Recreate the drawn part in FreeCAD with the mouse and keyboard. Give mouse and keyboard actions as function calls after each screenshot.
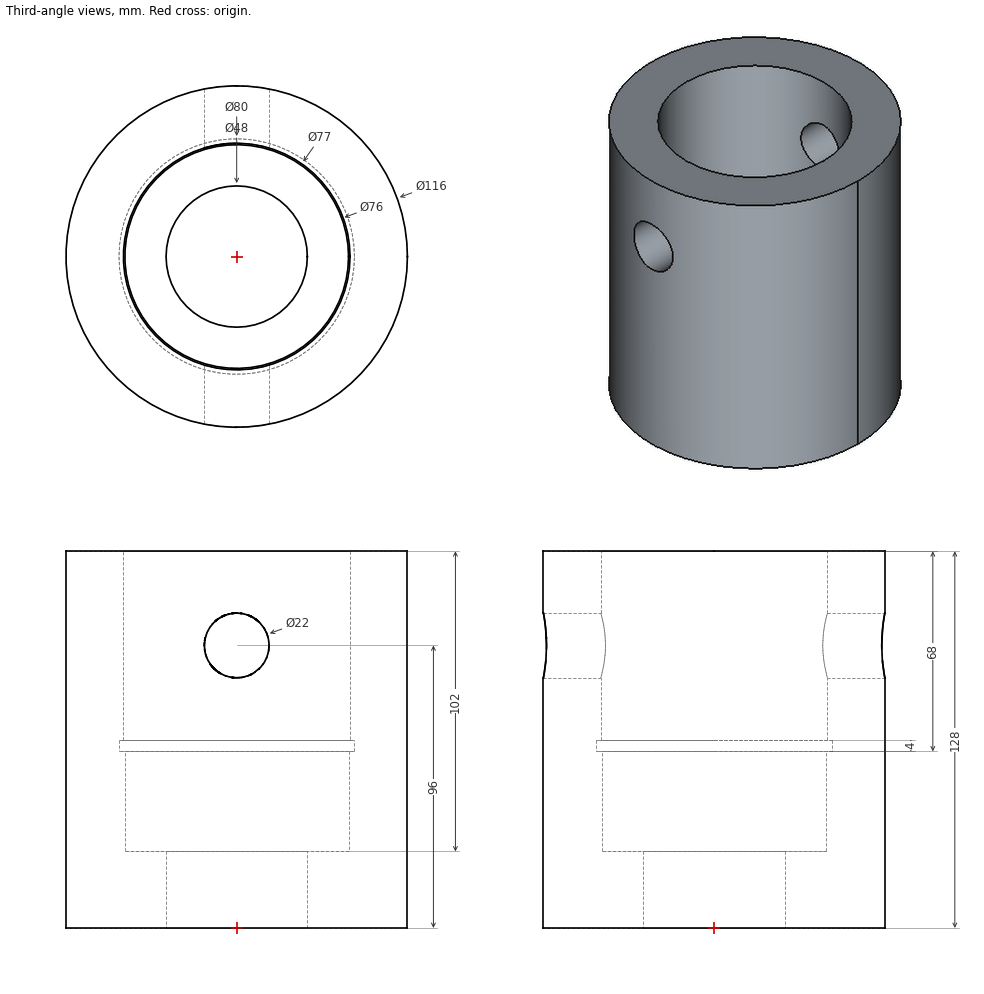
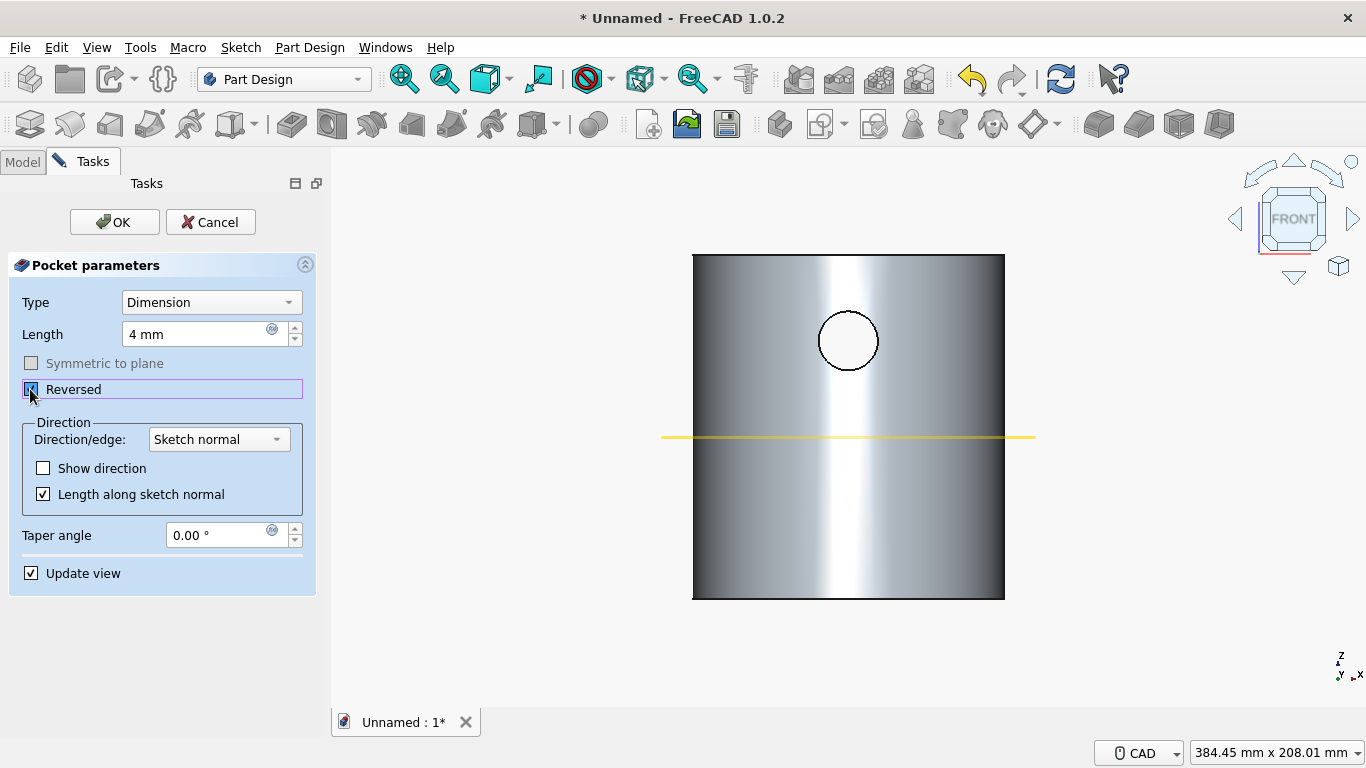
click(115, 222)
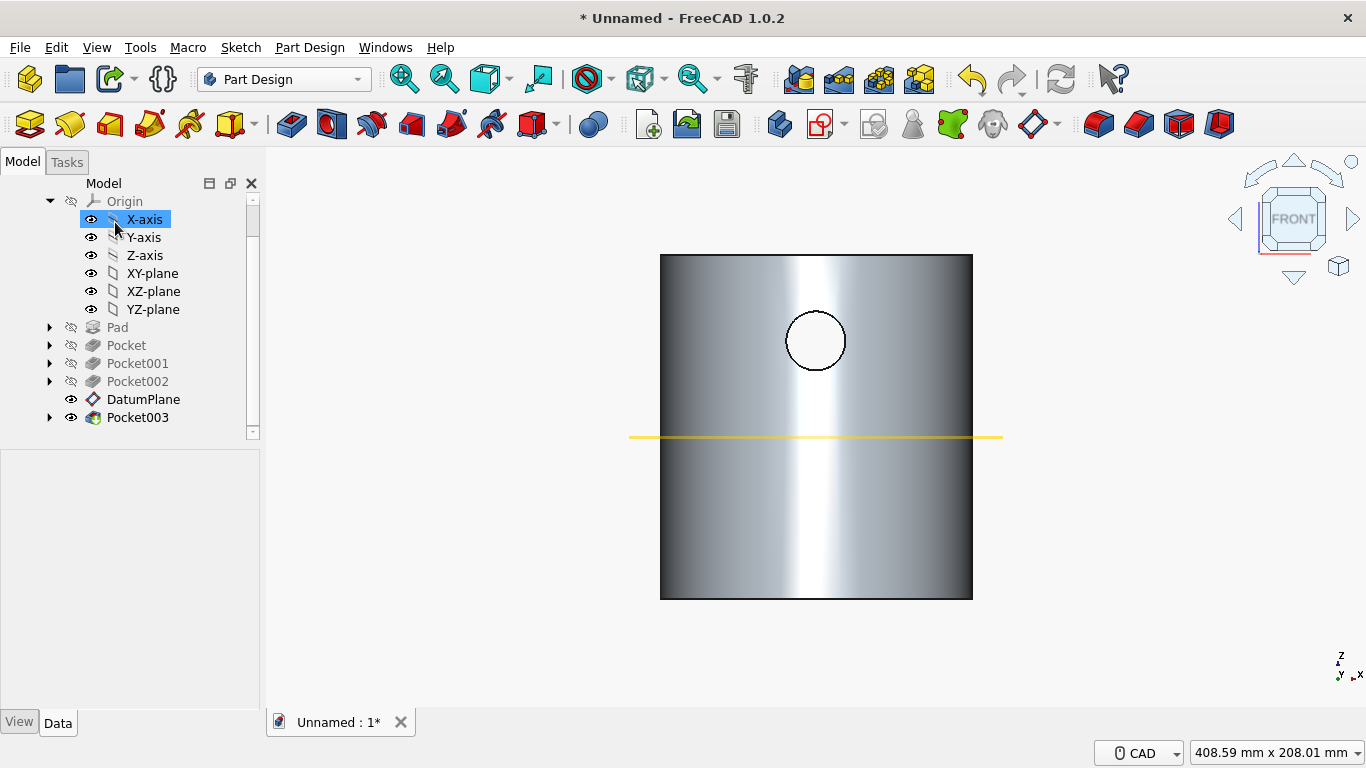
click(116, 399)
key(space)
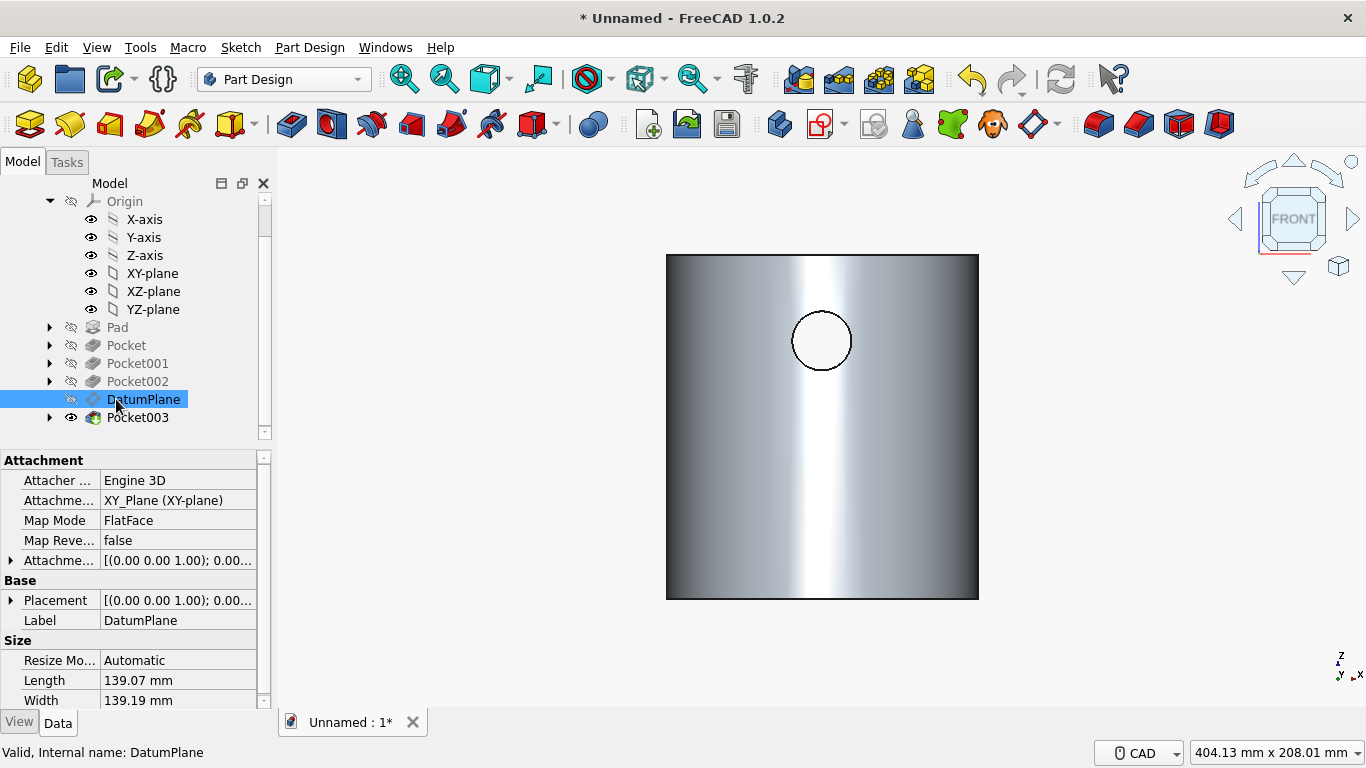
key(0)